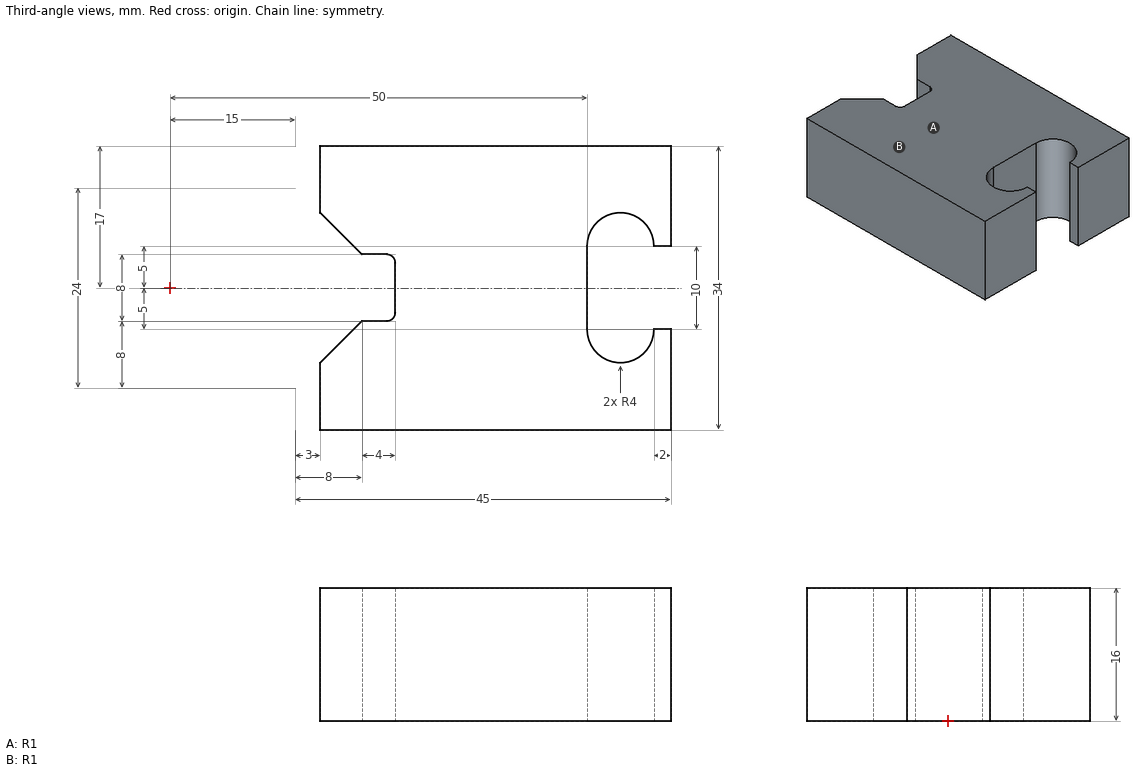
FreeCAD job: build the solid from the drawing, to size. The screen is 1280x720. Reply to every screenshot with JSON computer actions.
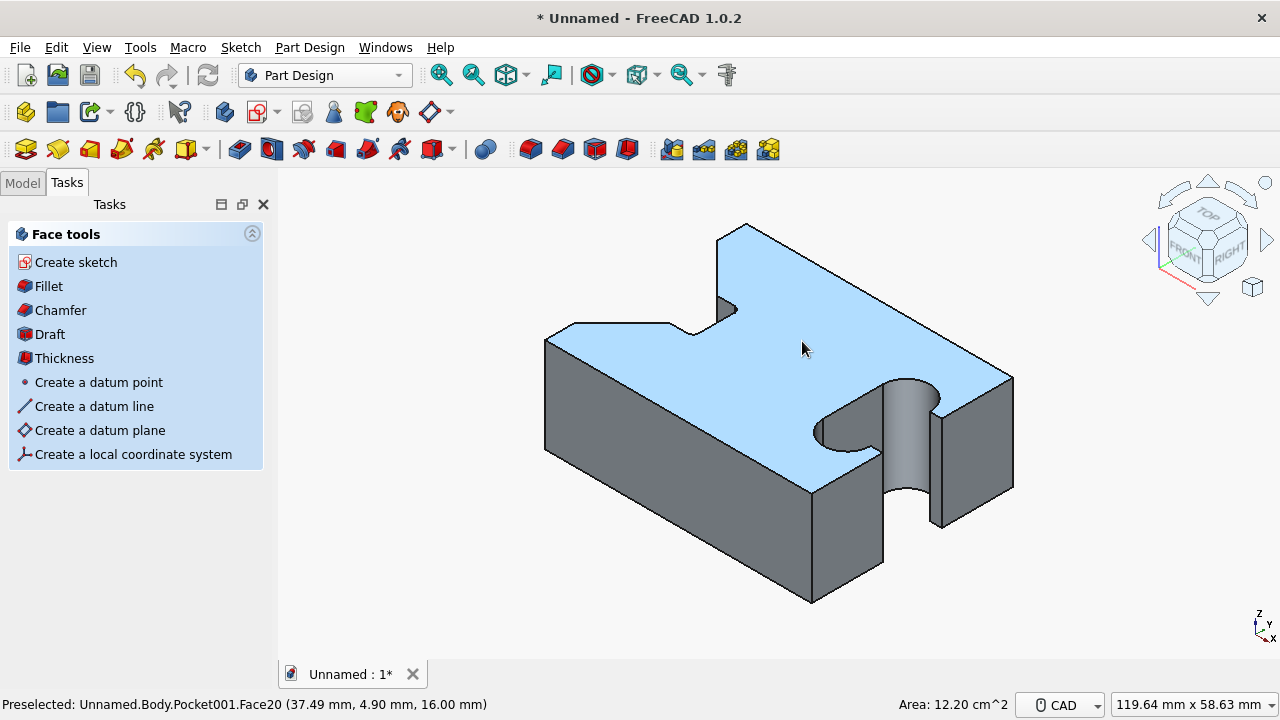
{"action": "left_click", "coordinate": [258, 112]}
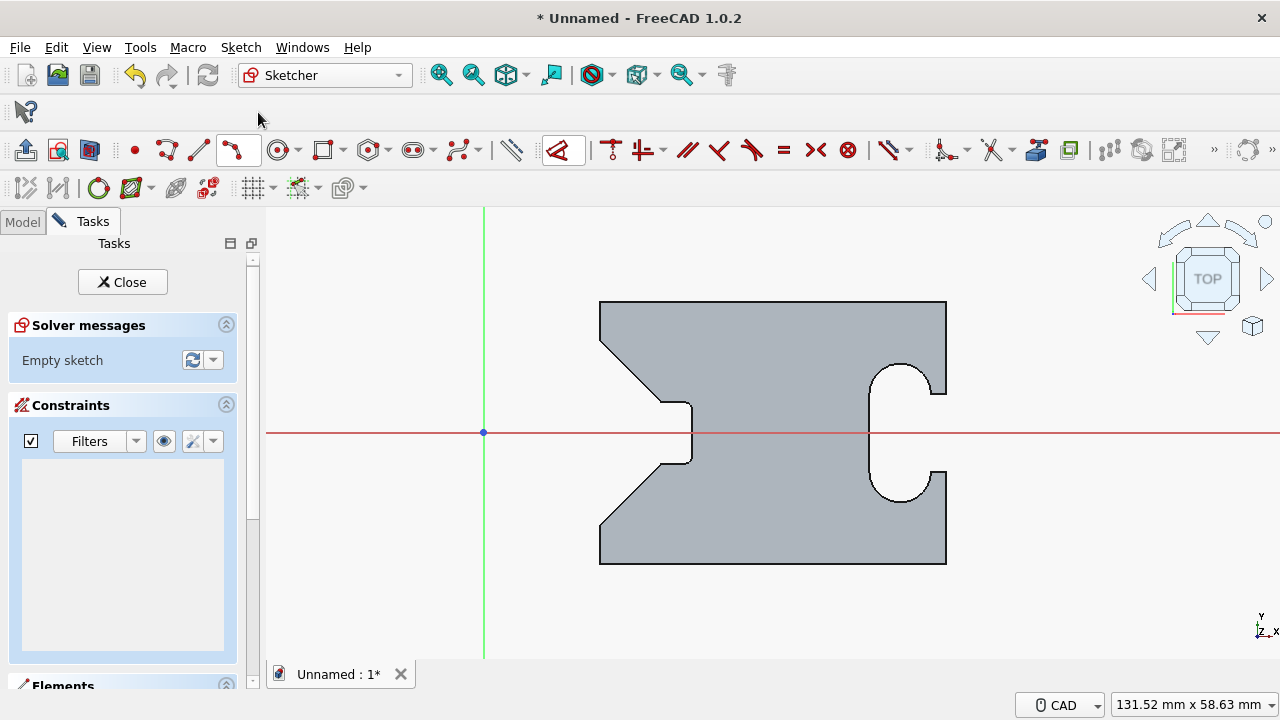
{"action": "left_click", "coordinate": [324, 150]}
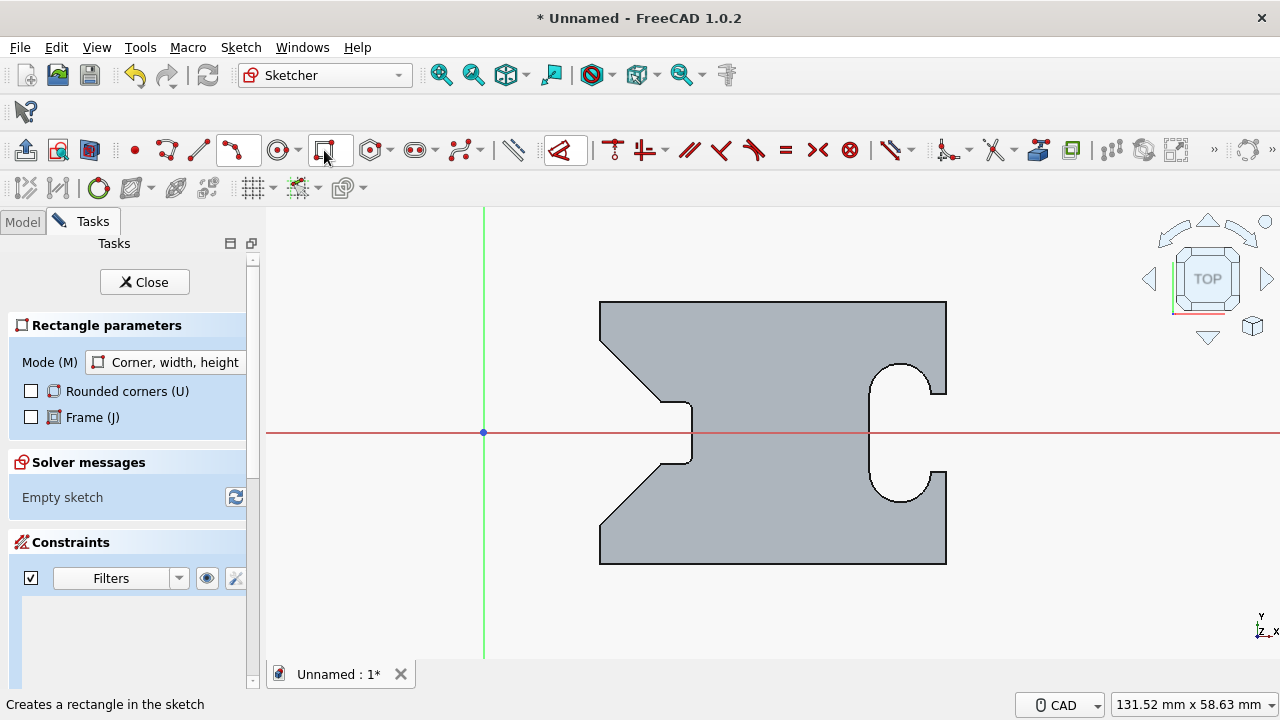
{"action": "left_click", "coordinate": [600, 302]}
{"action": "mouse_move", "coordinate": [623, 564]}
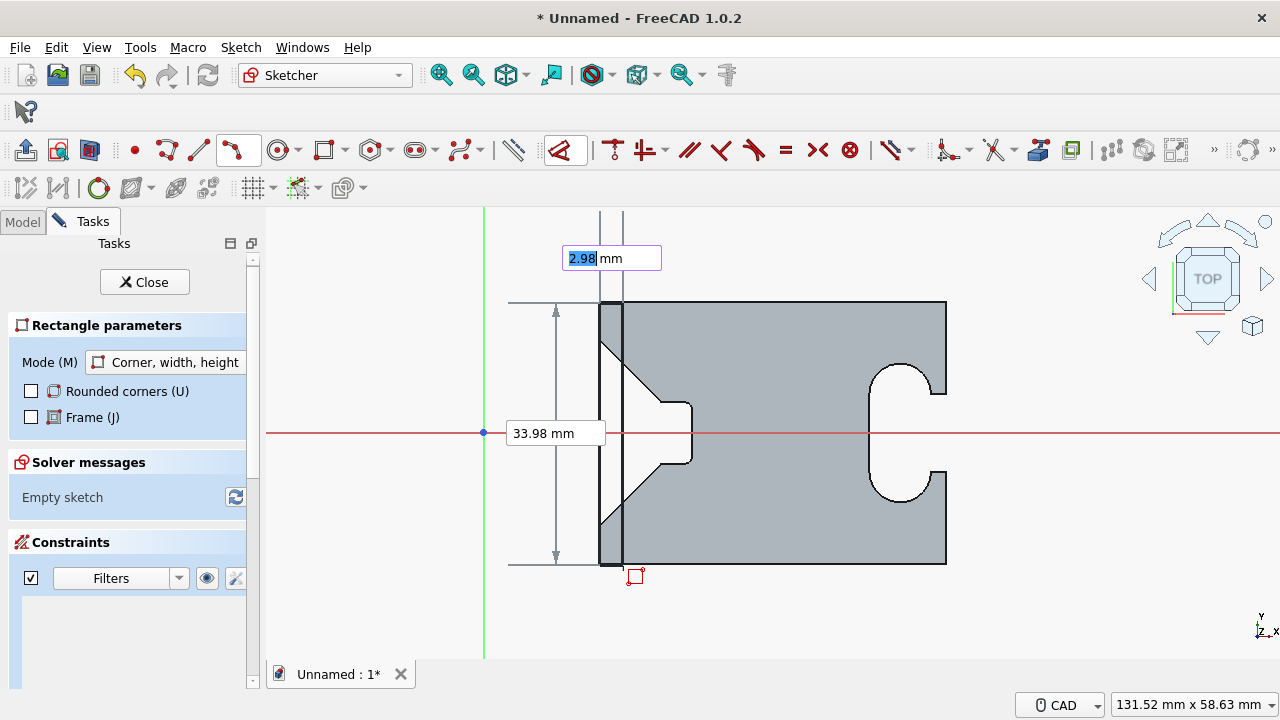
{"action": "type", "text": "3"}
{"action": "key", "text": "Tab"}
{"action": "type", "text": "34"}
{"action": "key", "text": "Return"}
{"action": "key", "text": "Escape"}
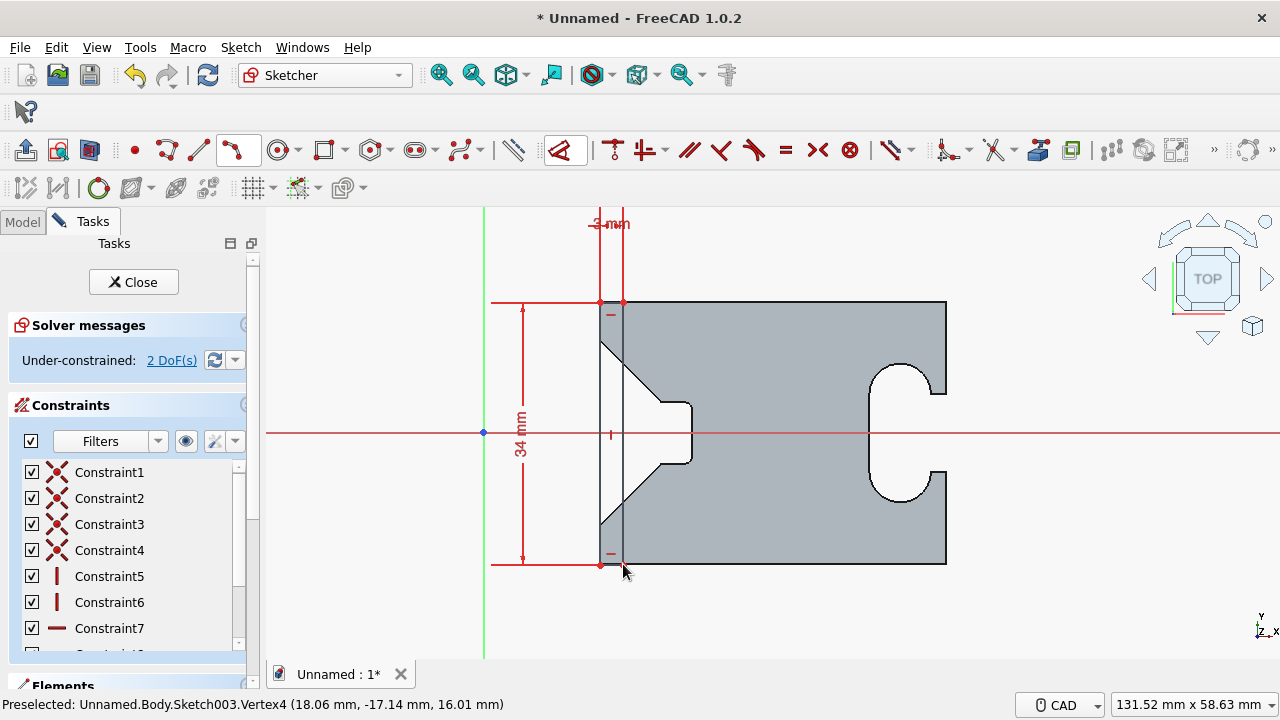
{"action": "left_click", "coordinate": [600, 303]}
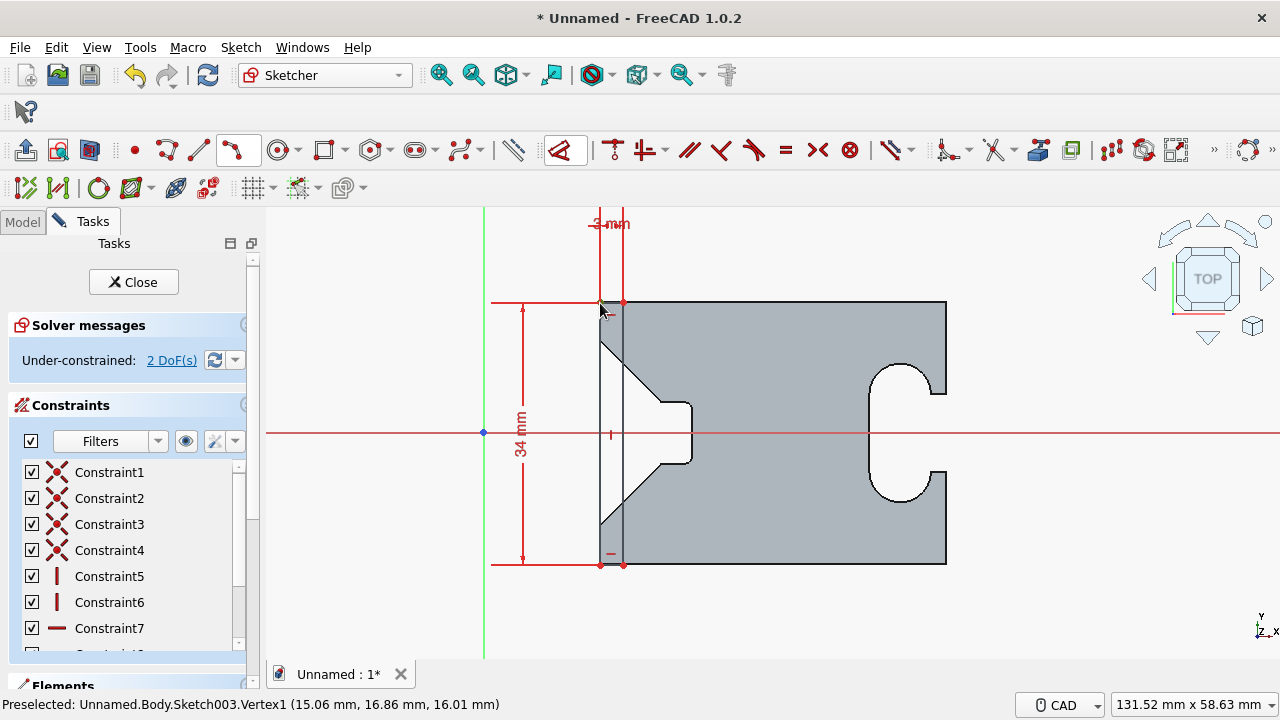
{"action": "left_click", "coordinate": [582, 150]}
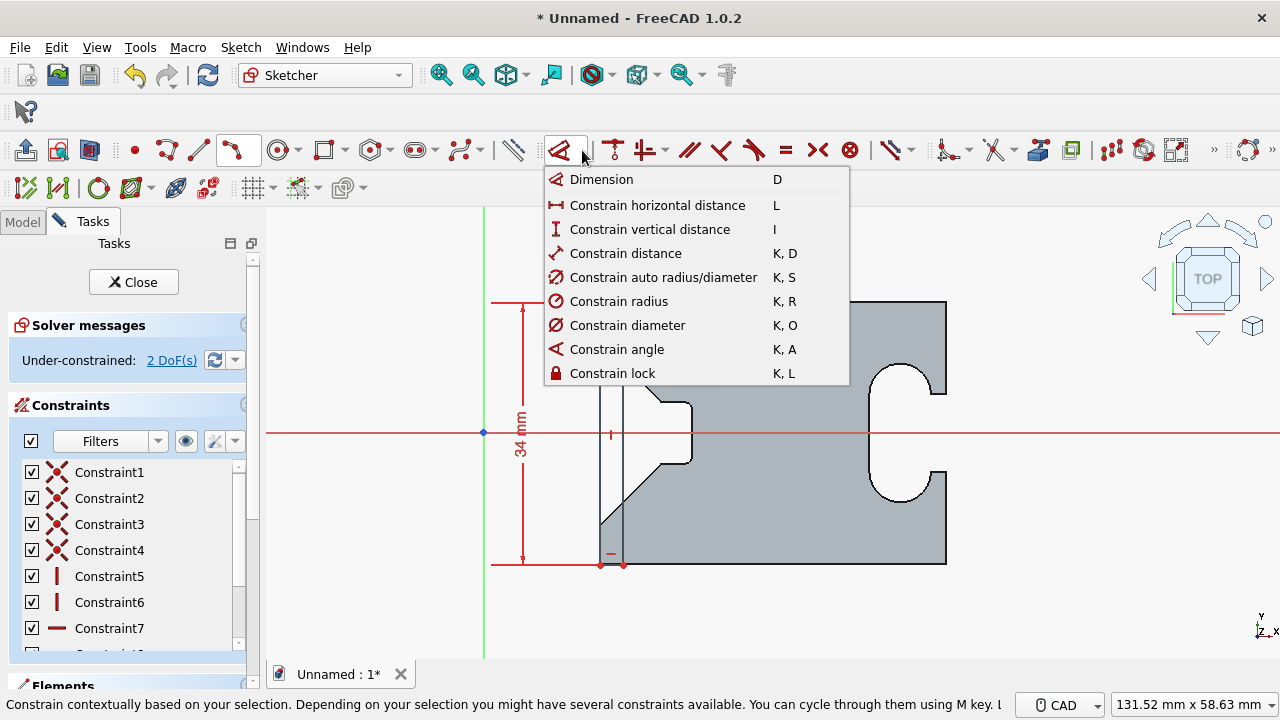
{"action": "left_click", "coordinate": [697, 205]}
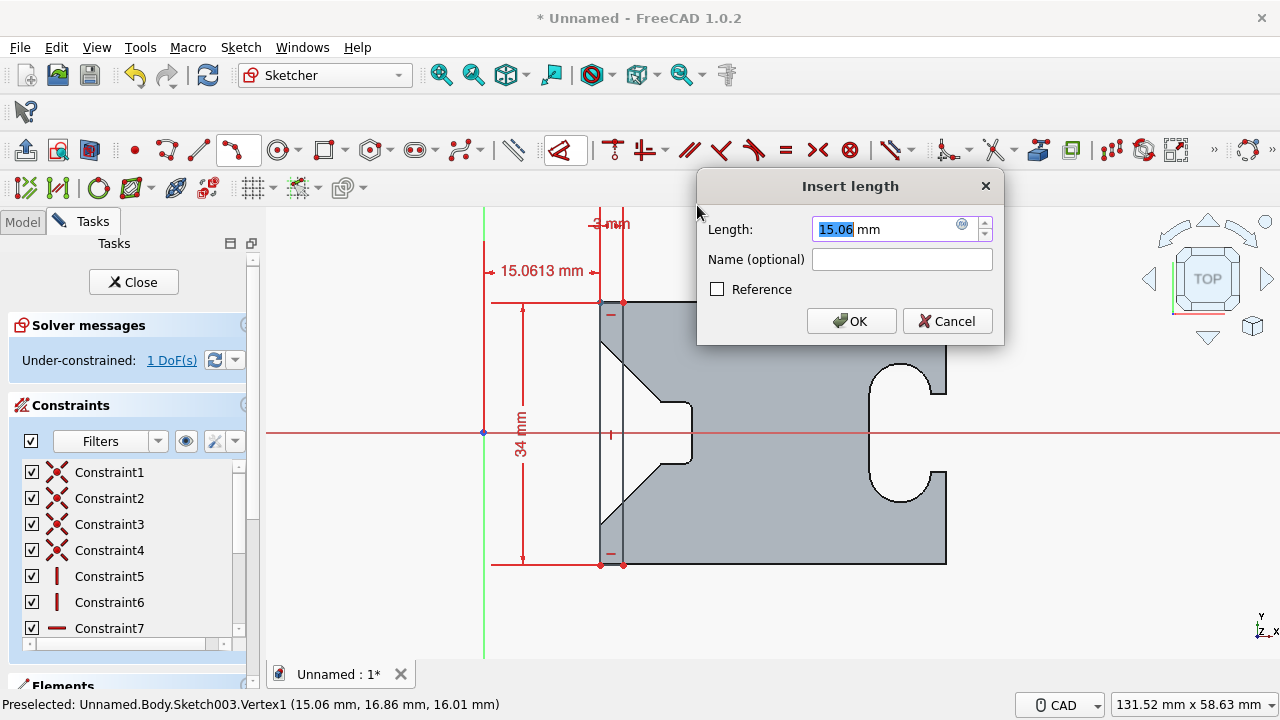
{"action": "type", "text": "15"}
{"action": "key", "text": "Return"}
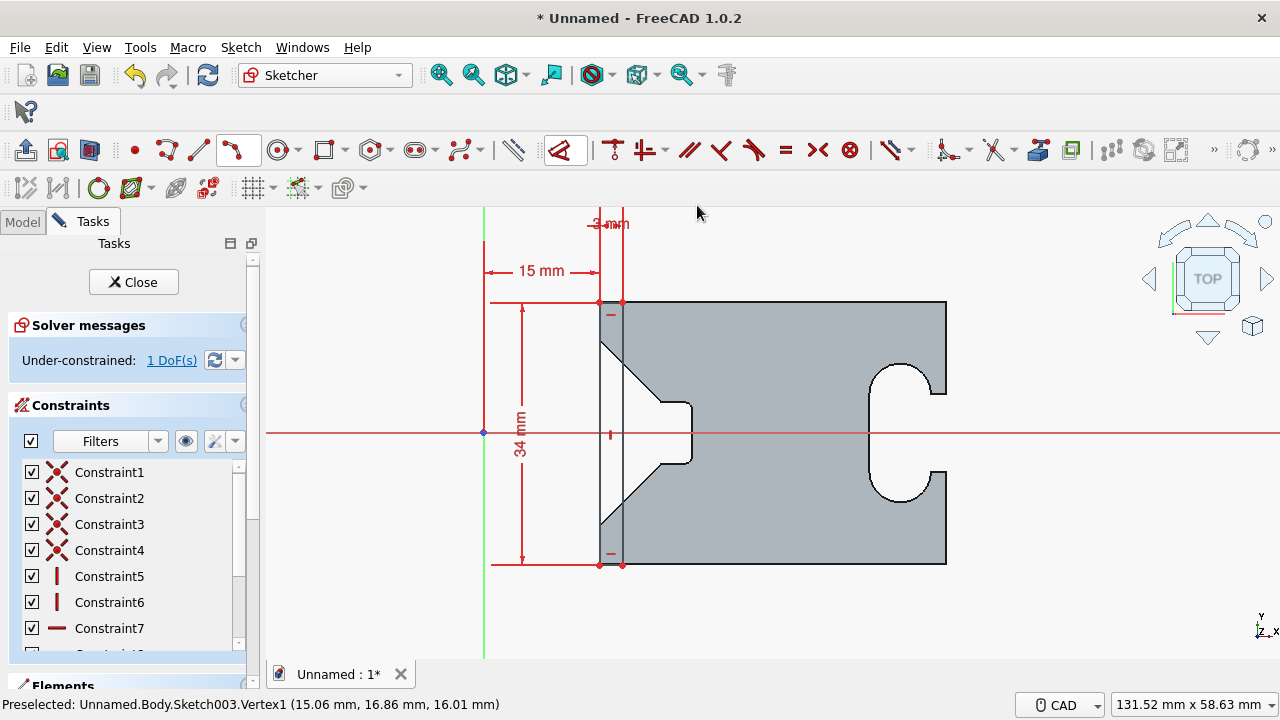
{"action": "left_click", "coordinate": [600, 303]}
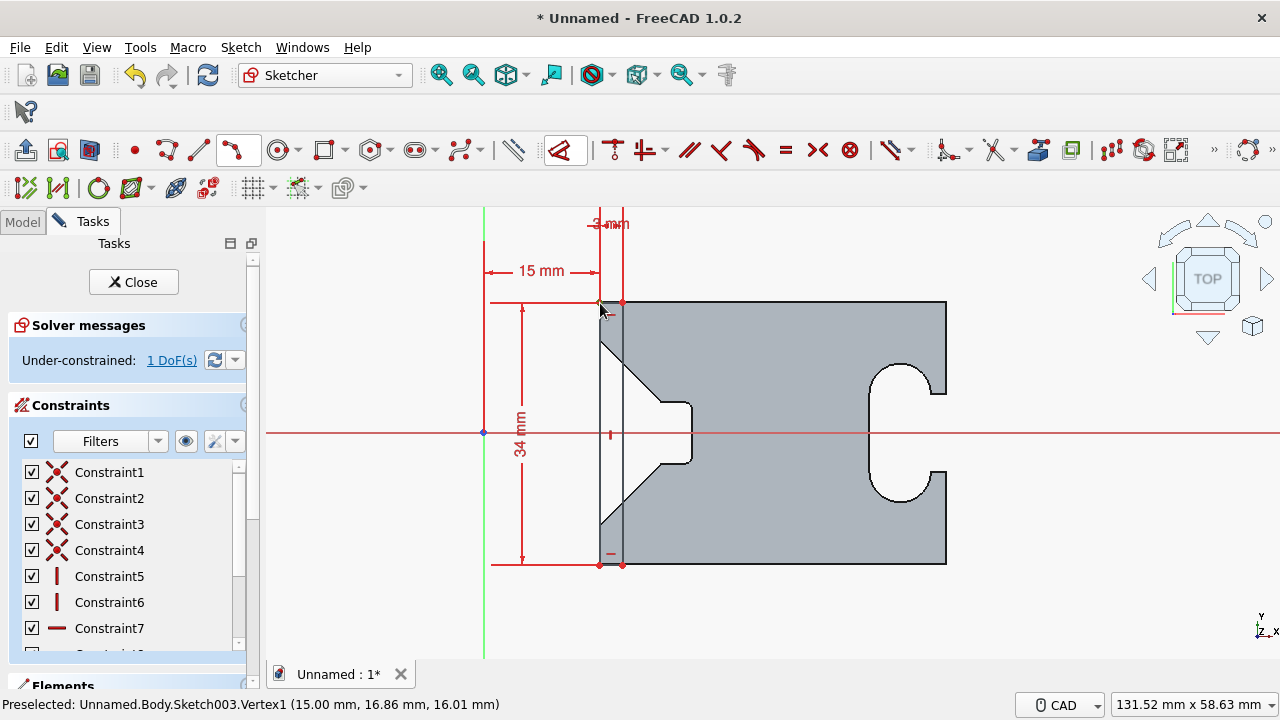
{"action": "key", "text": "i"}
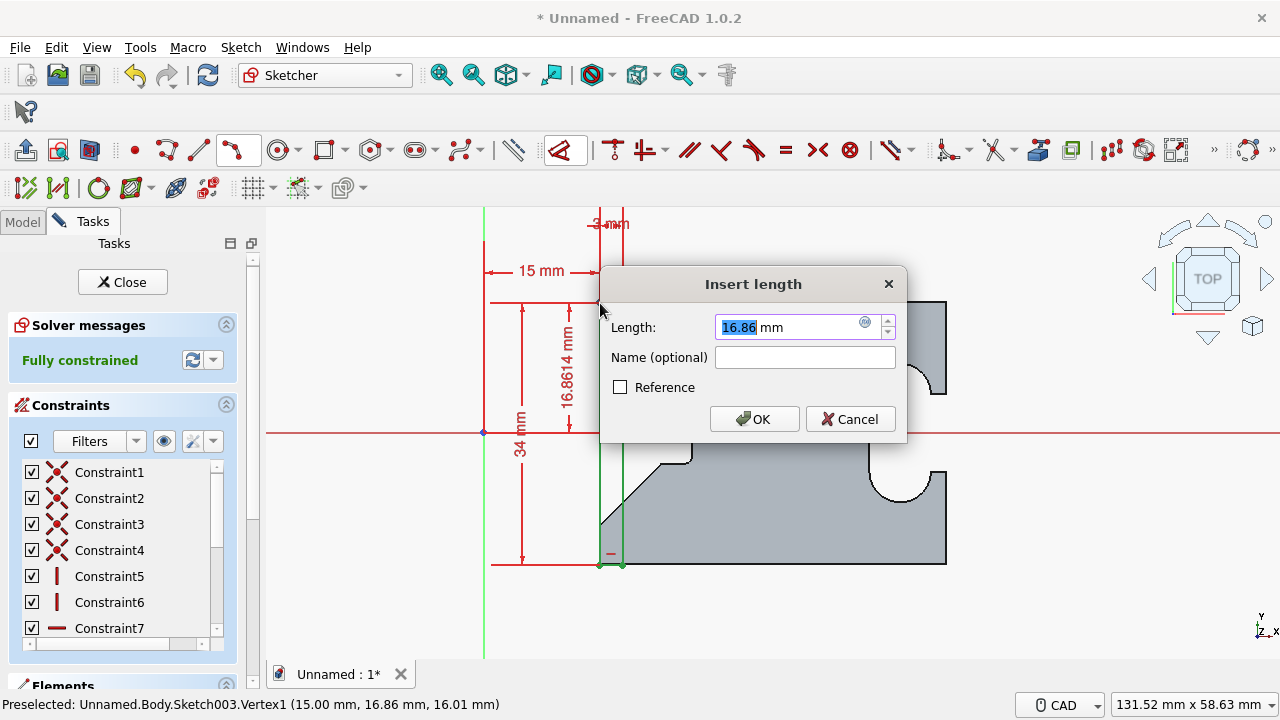
{"action": "type", "text": "17"}
{"action": "key", "text": "Return"}